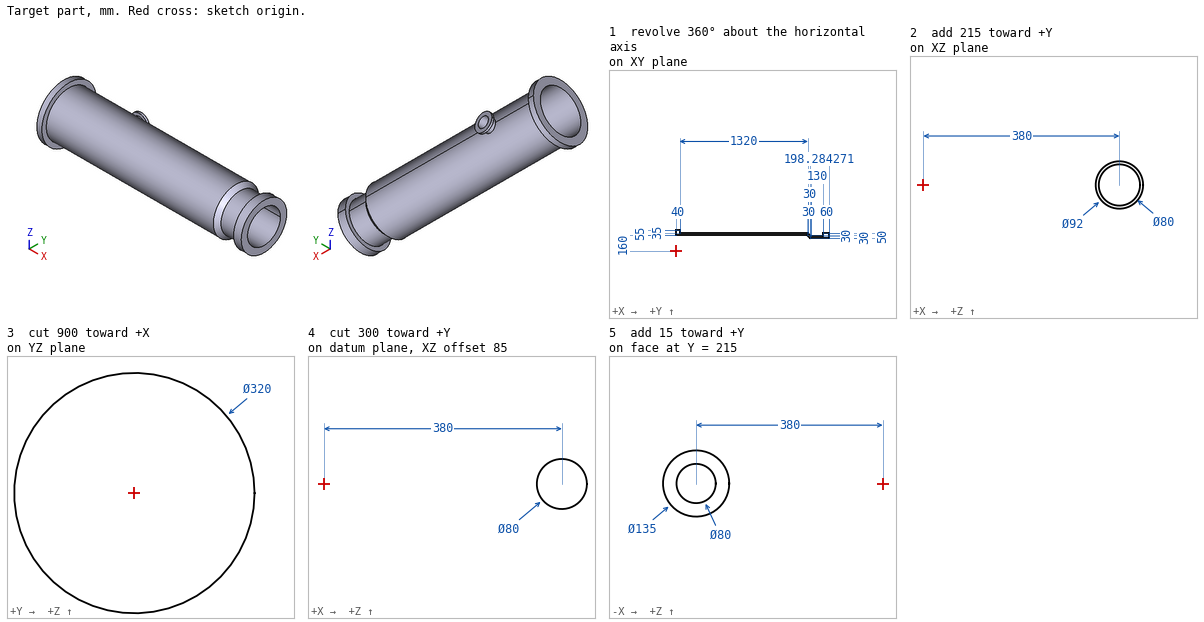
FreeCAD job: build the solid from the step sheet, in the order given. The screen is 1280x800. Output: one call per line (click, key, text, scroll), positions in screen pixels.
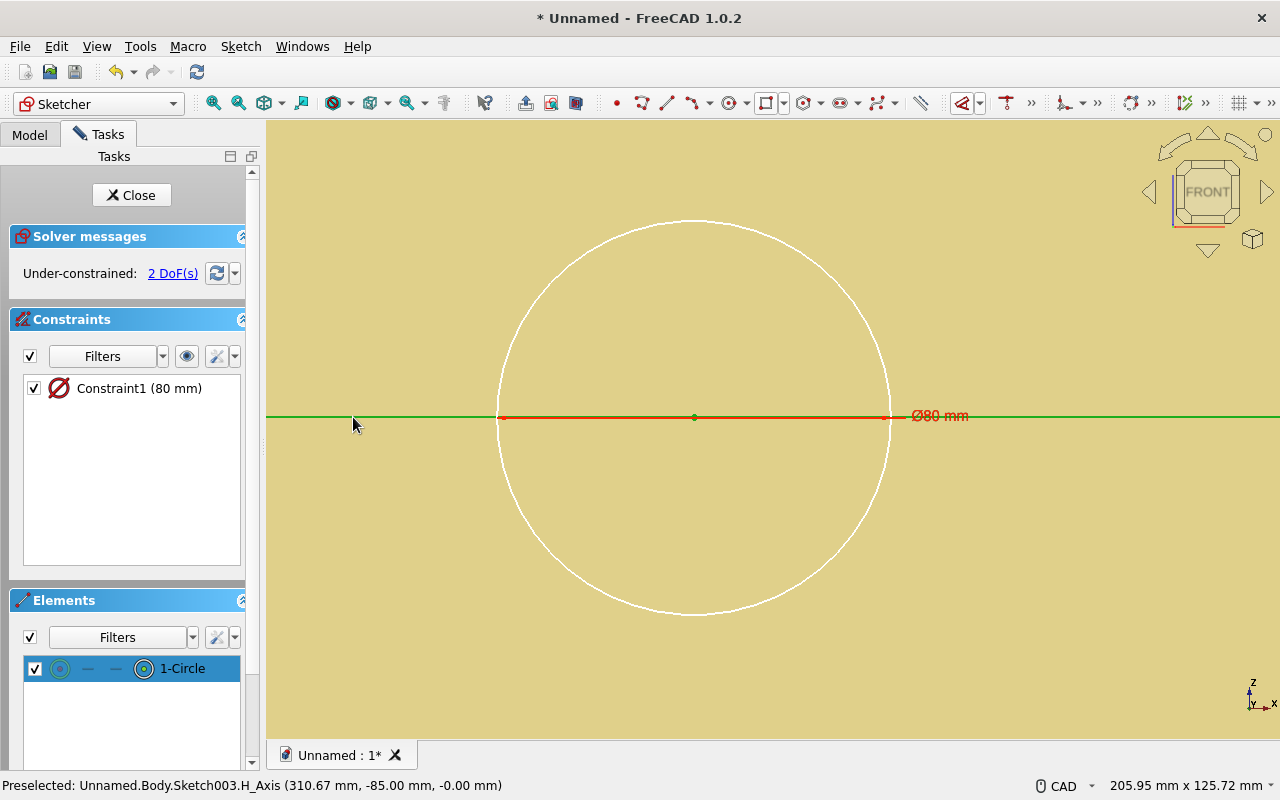
key(c)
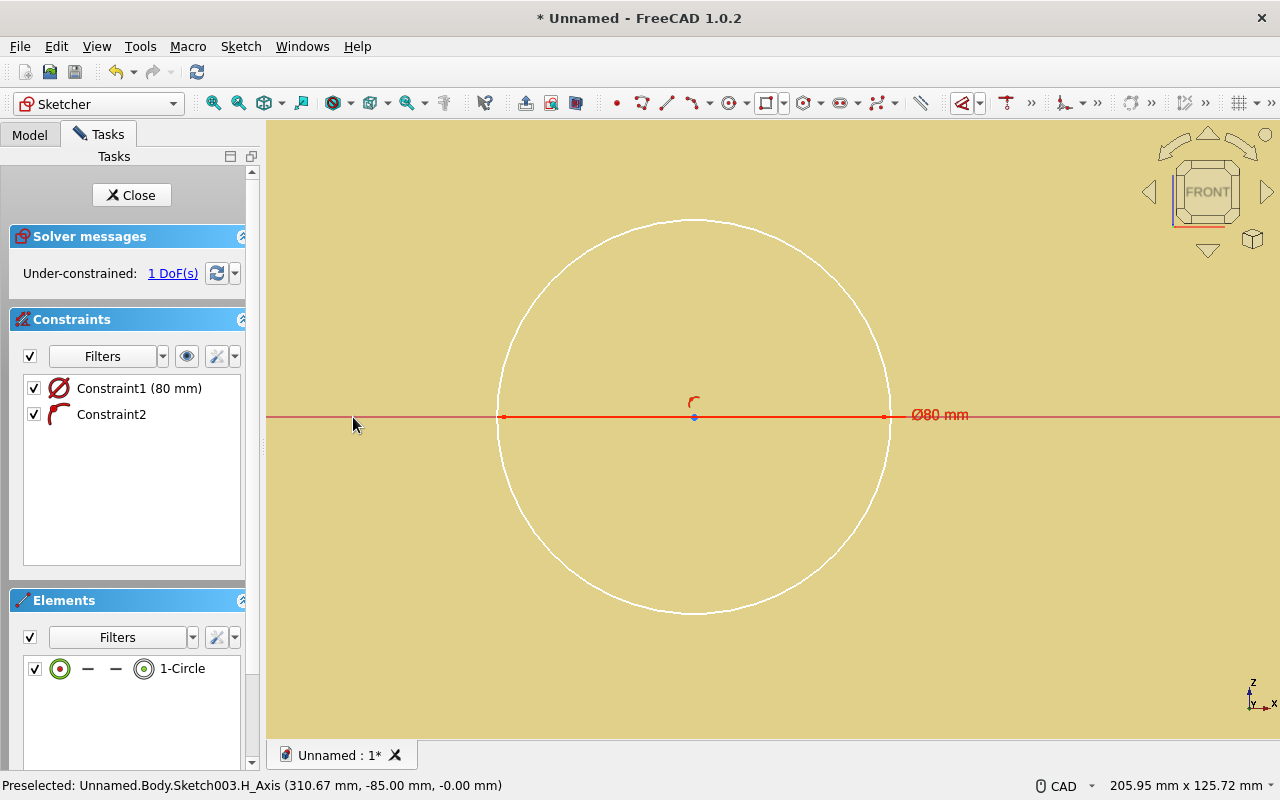
click(694, 417)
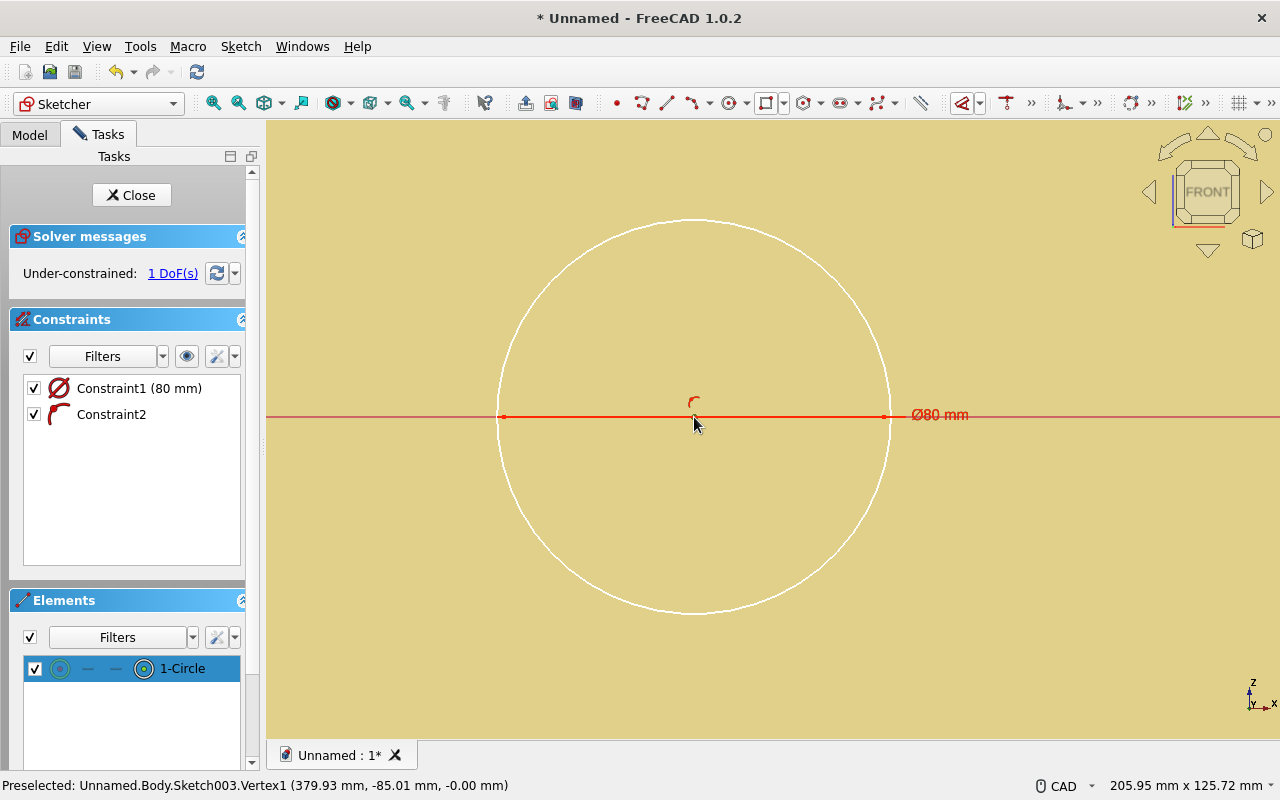
key(l)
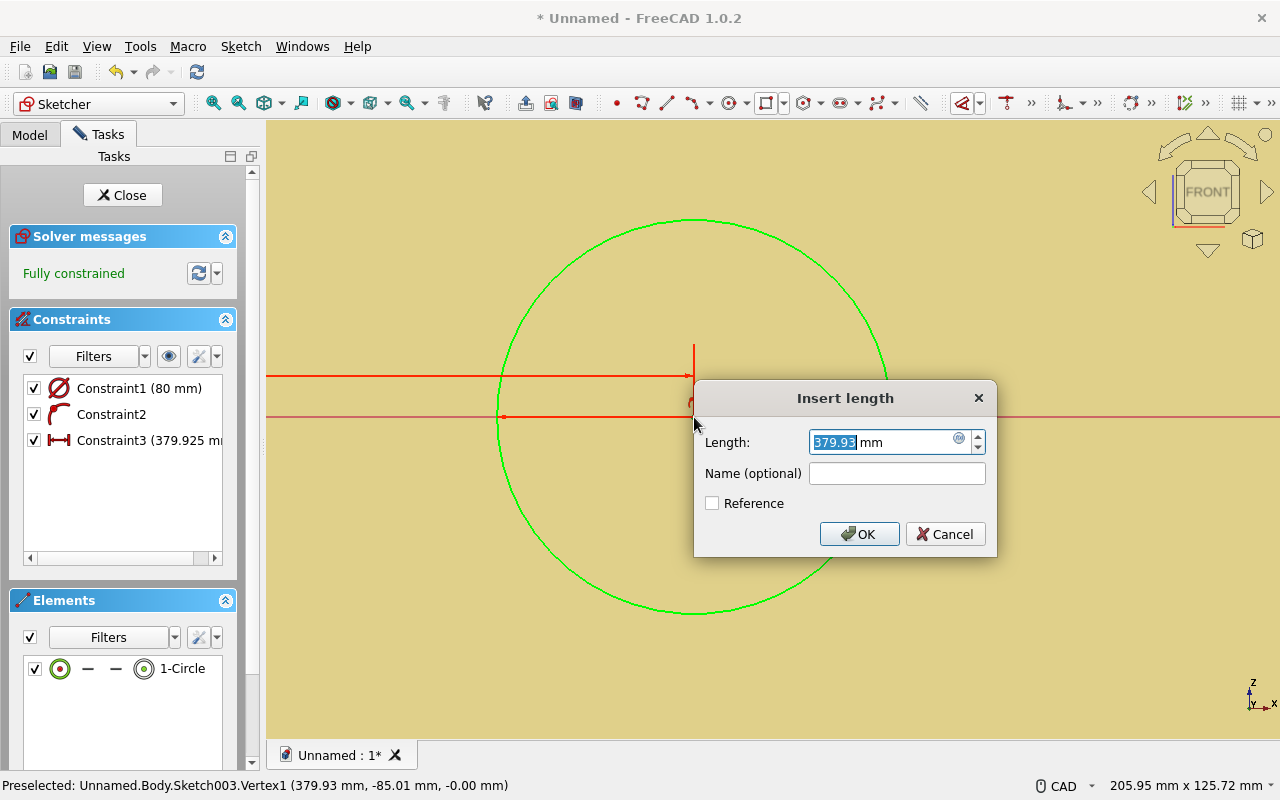
text(380)
key(Return)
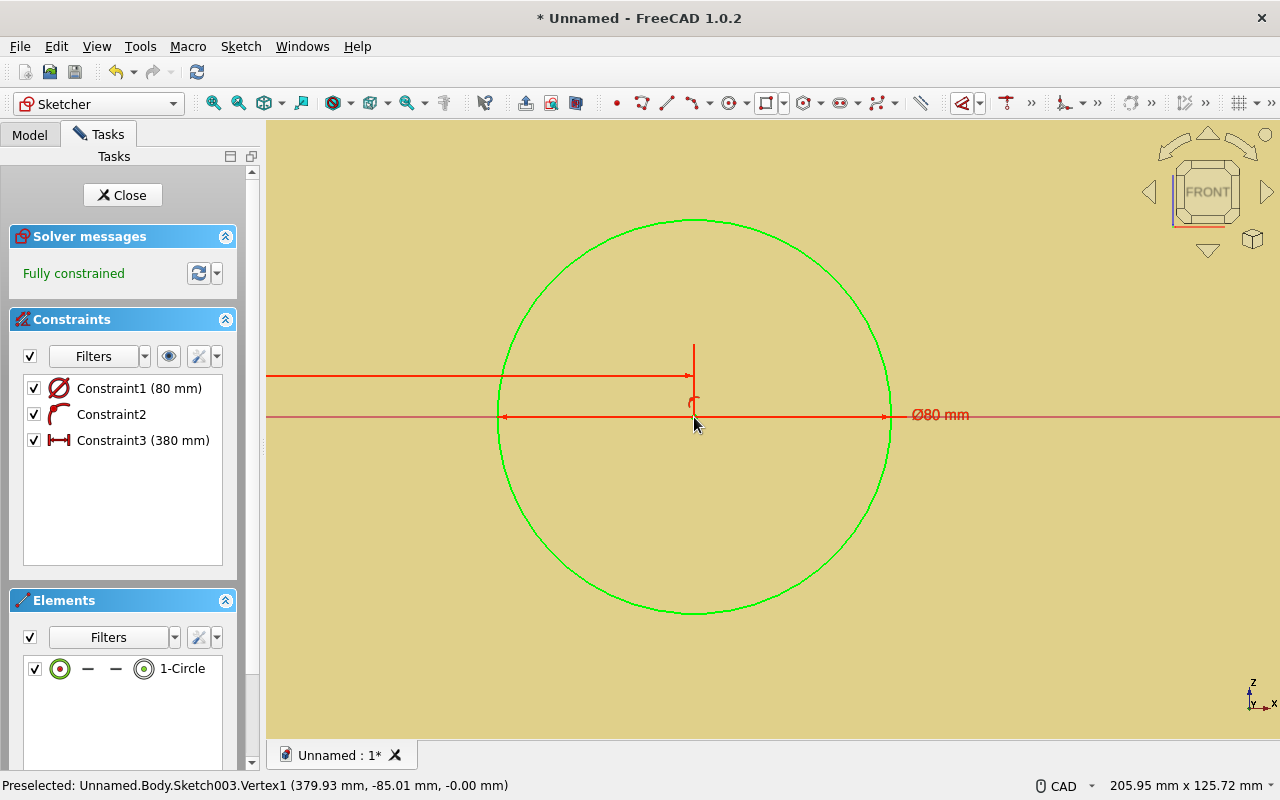
click(123, 195)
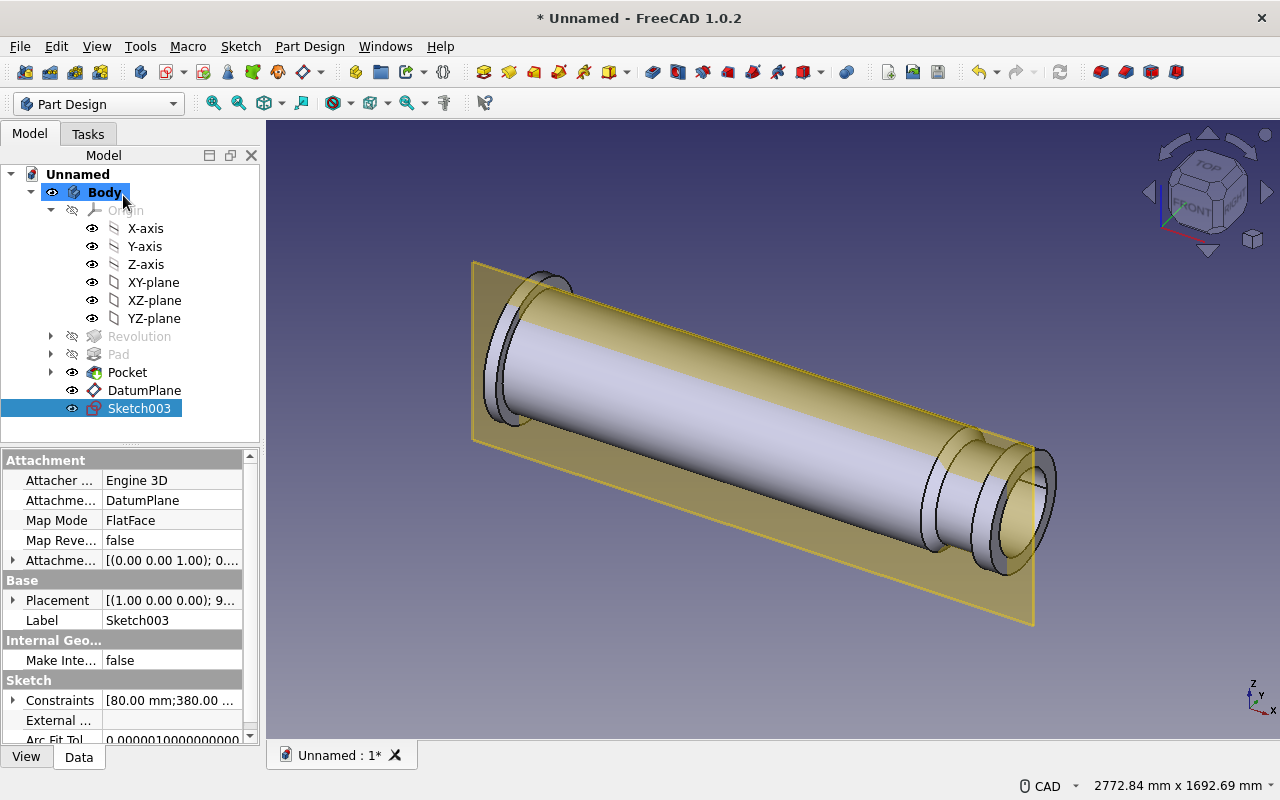
click(653, 72)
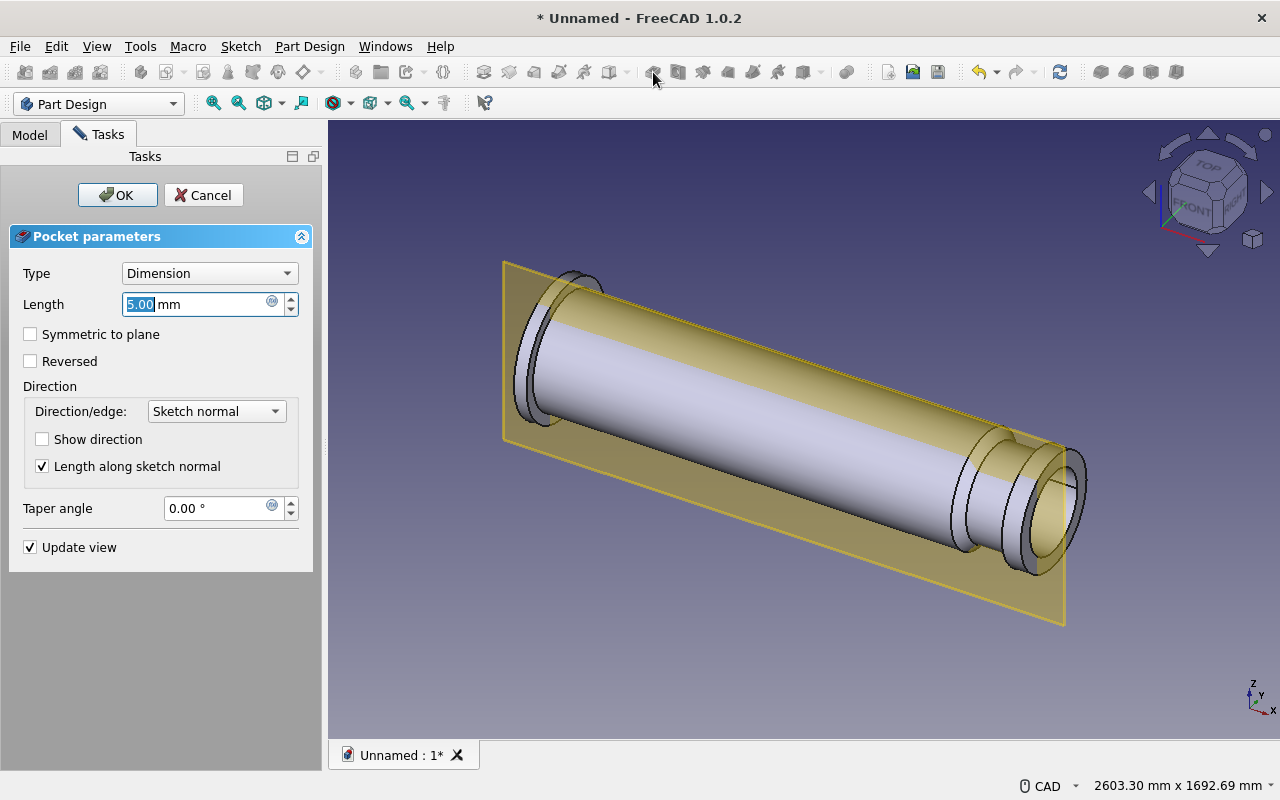
text(300)
key(Tab)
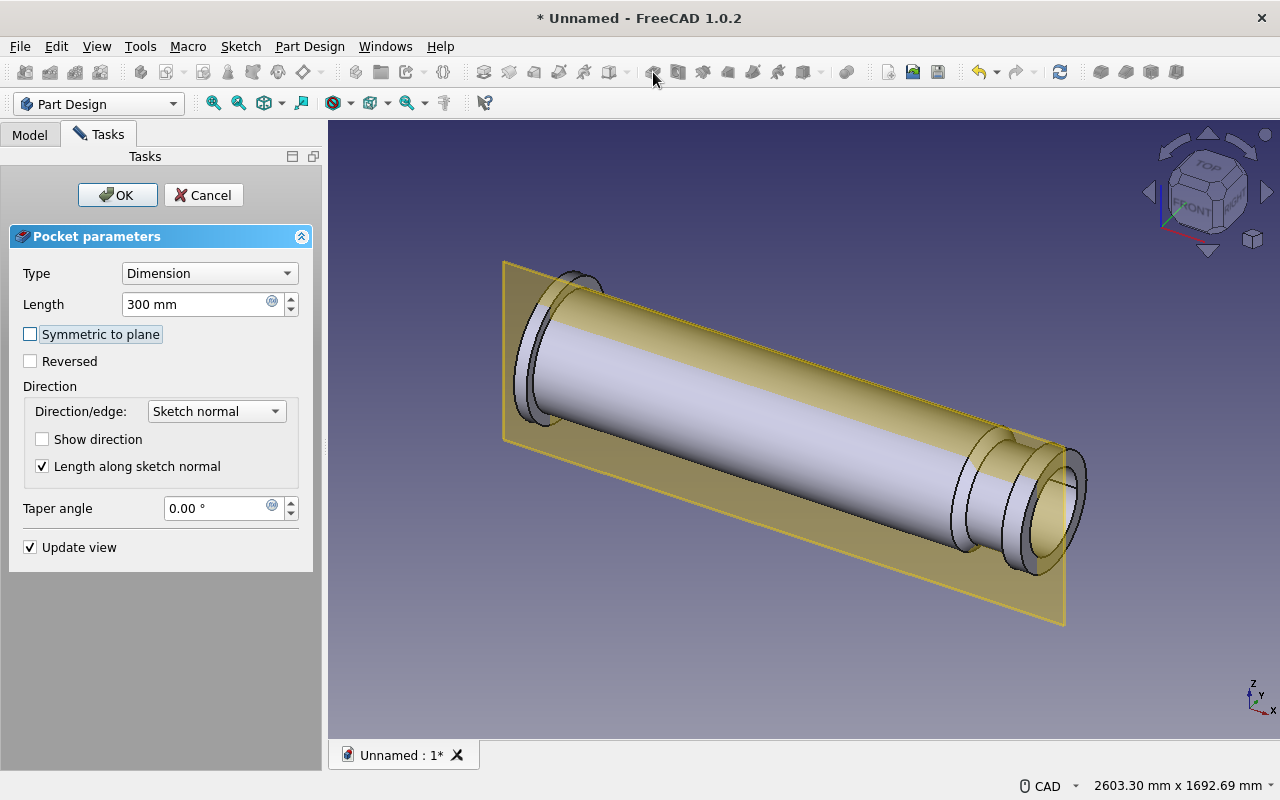
click(118, 195)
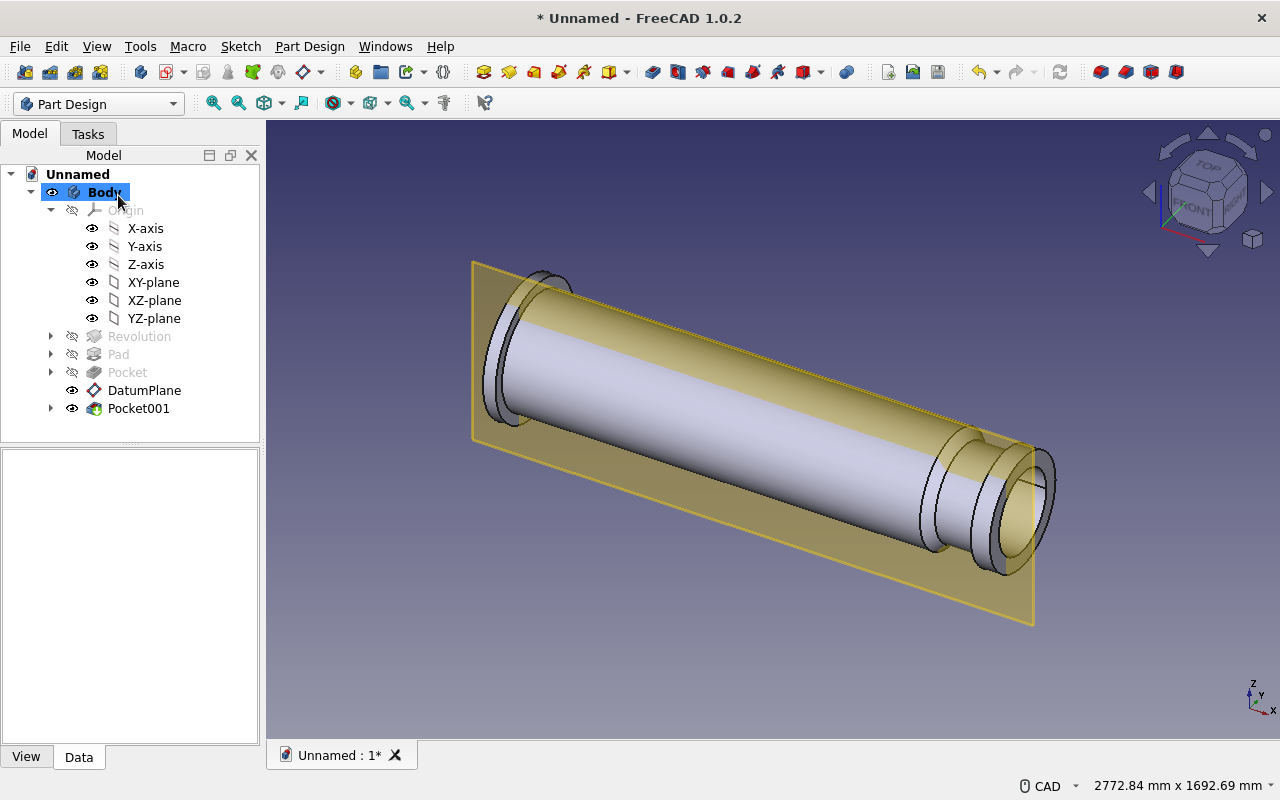
click(117, 390)
key(space)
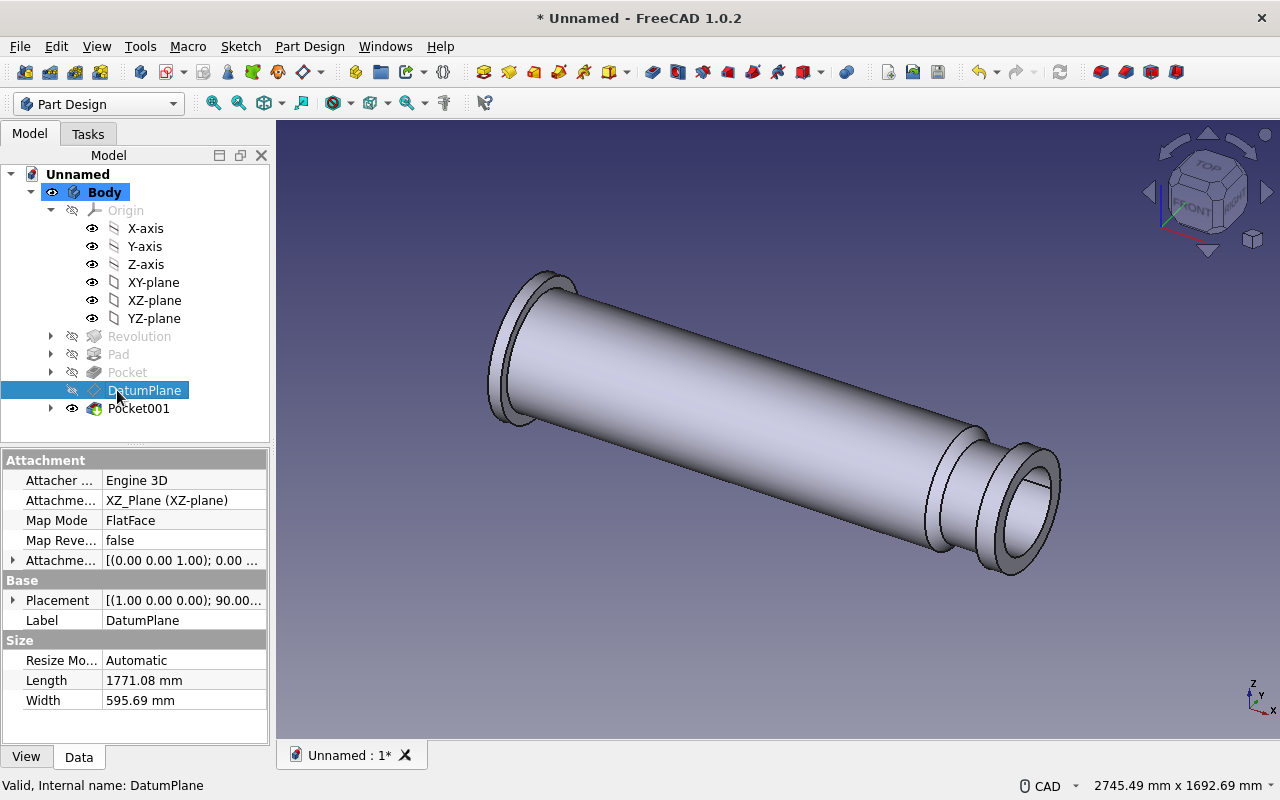
key(4)